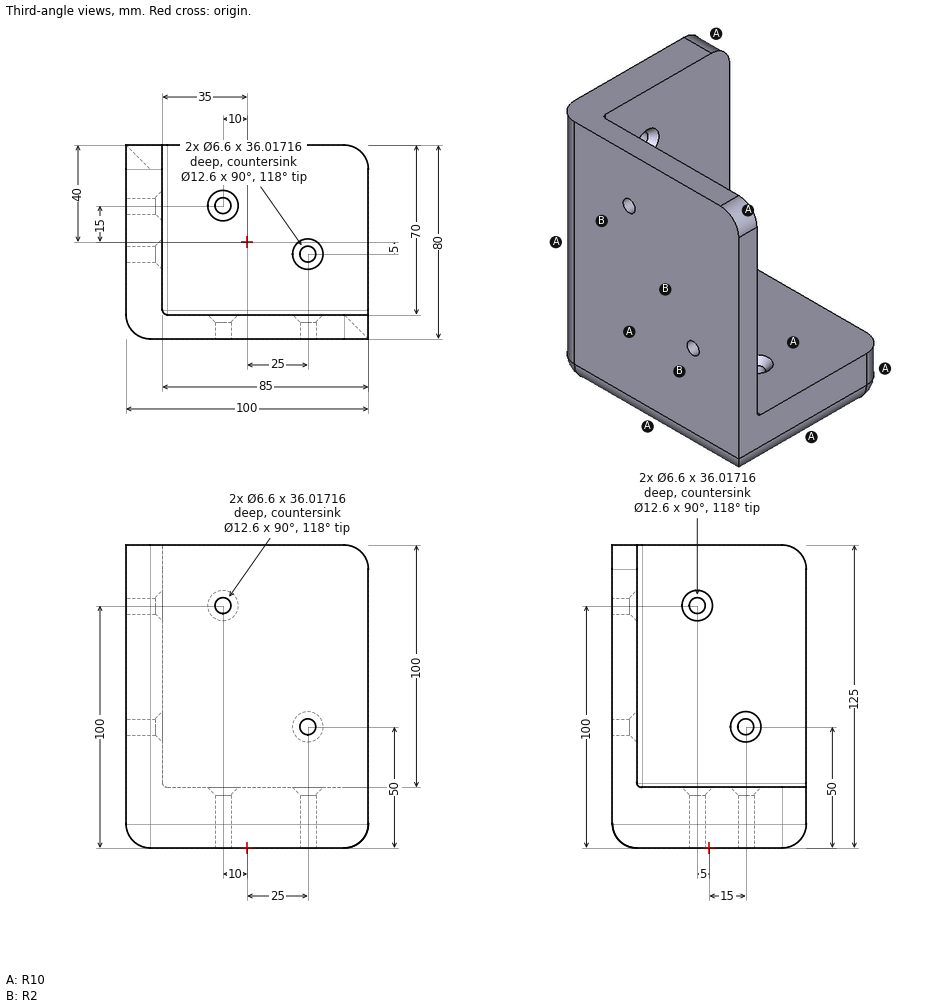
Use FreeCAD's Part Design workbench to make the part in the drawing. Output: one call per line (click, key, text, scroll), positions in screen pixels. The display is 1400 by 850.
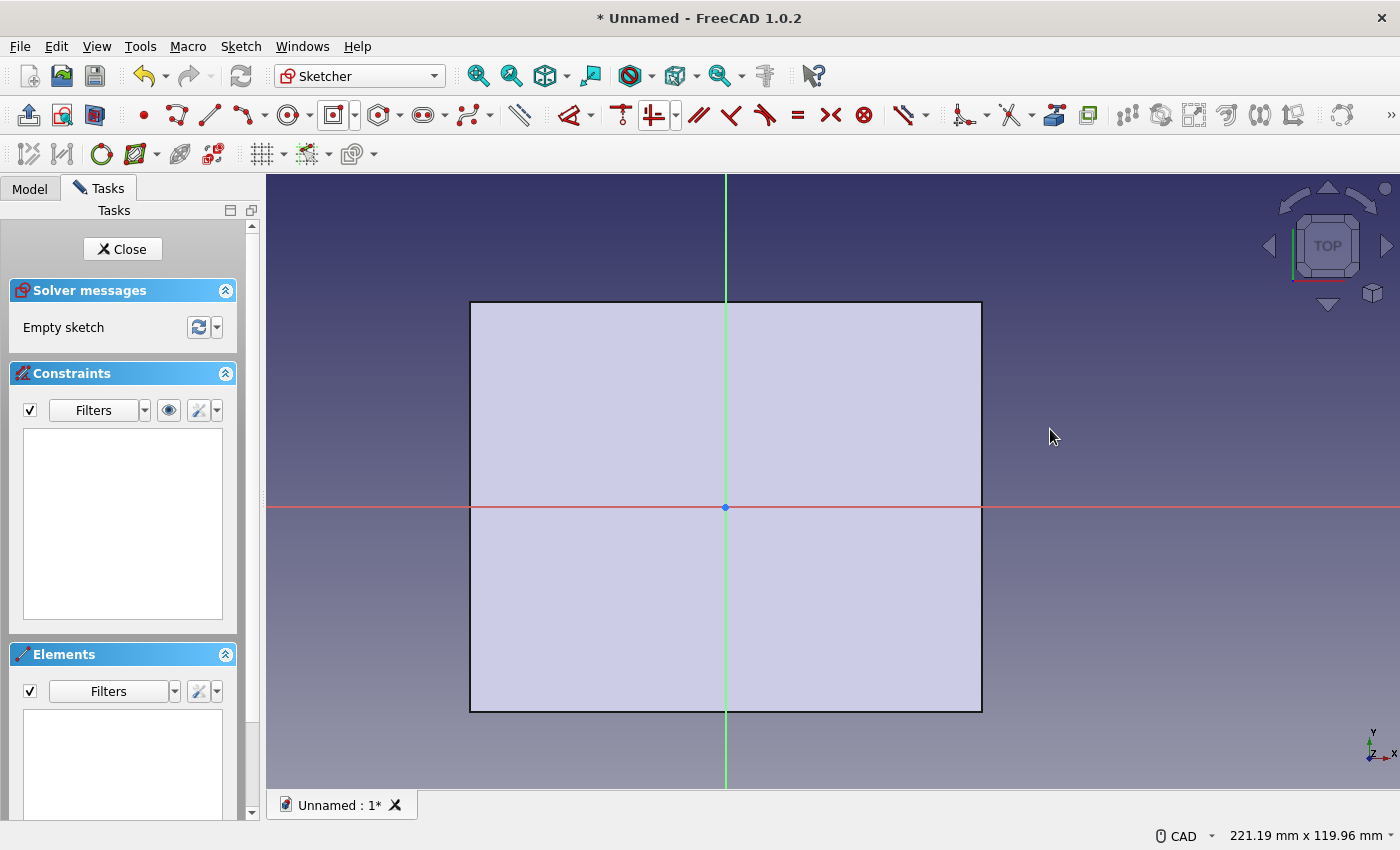
key(g)
key(r)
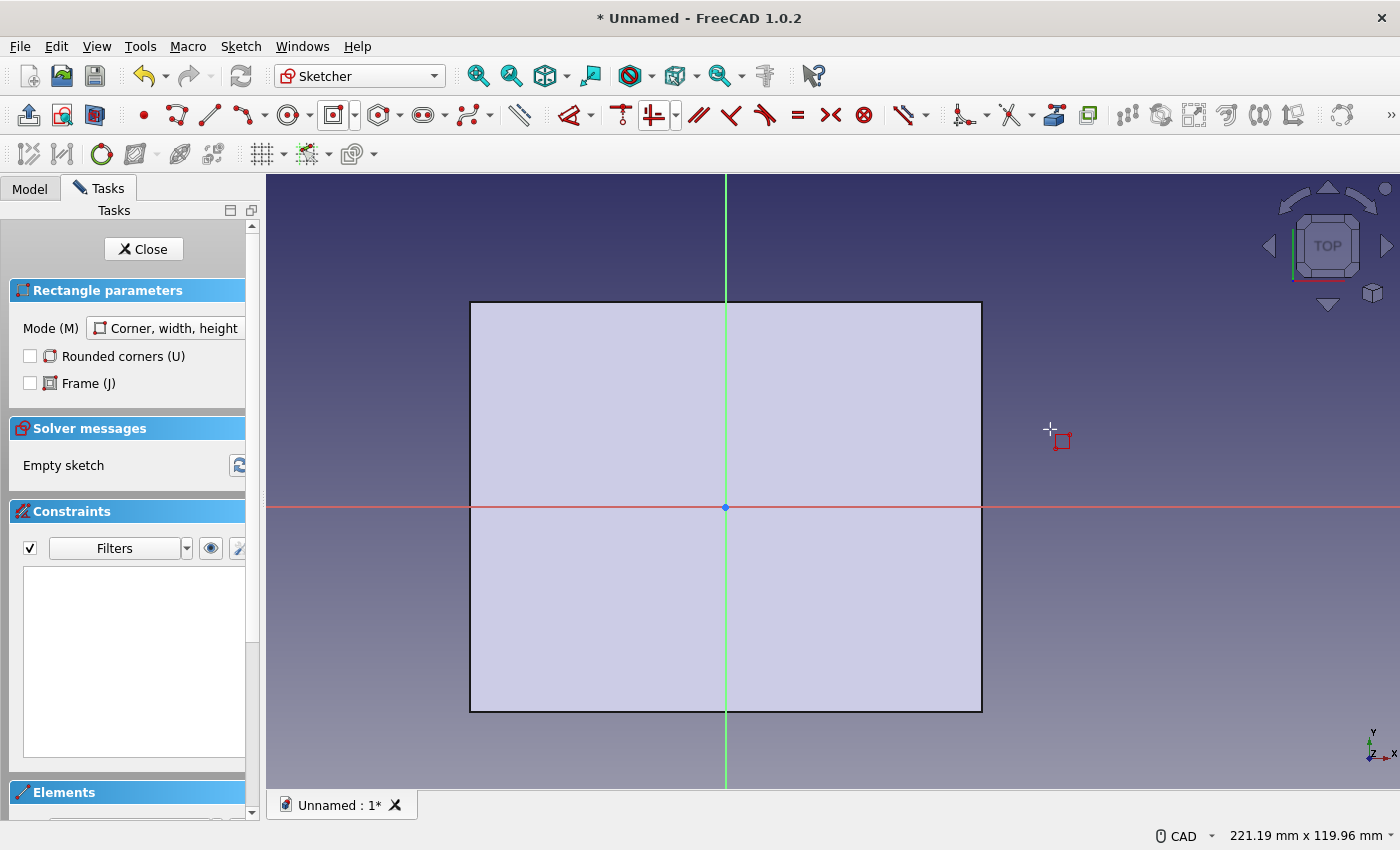
click(546, 302)
move(982, 661)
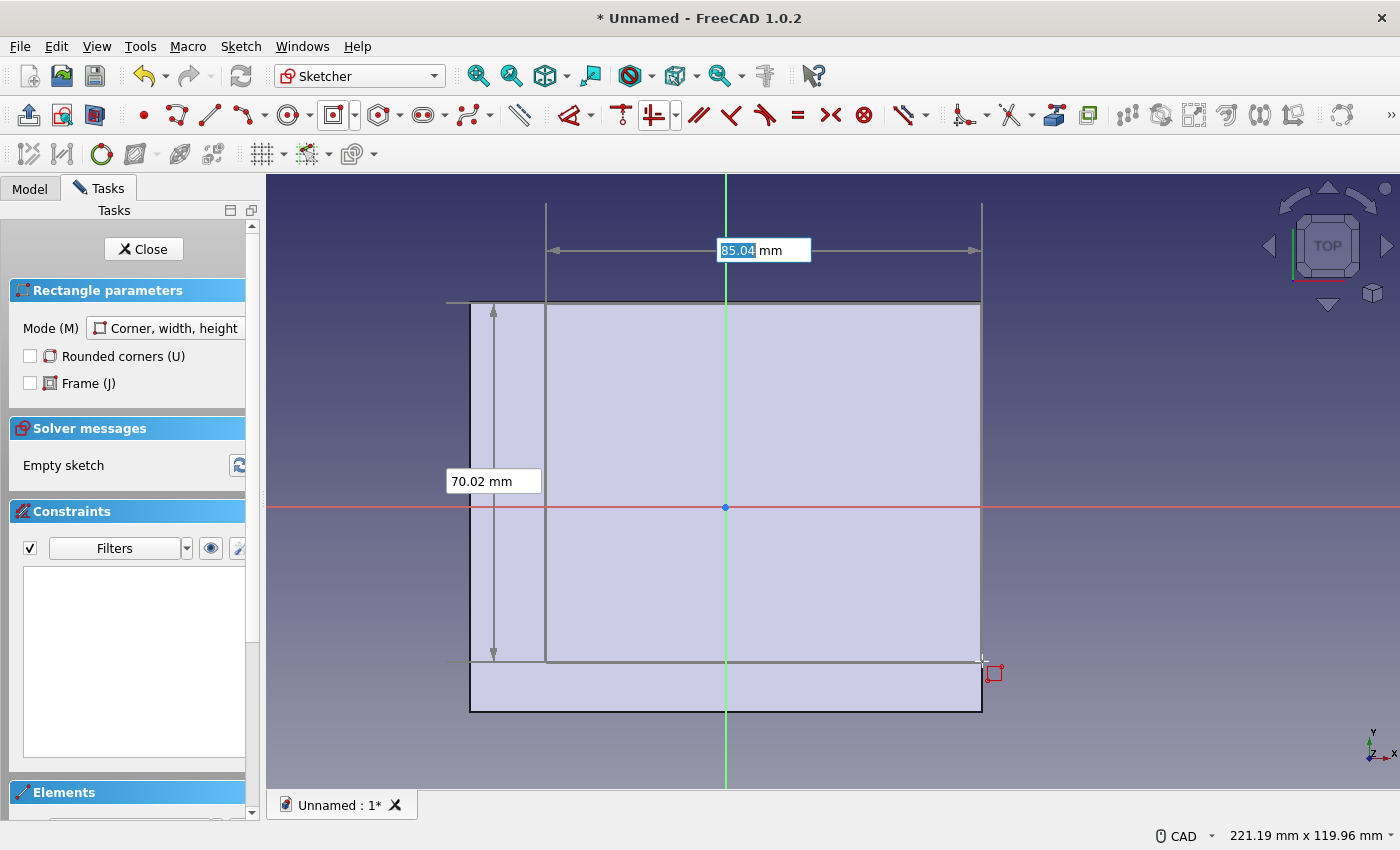
text(85)
key(Tab)
text(70)
key(Return)
key(Escape)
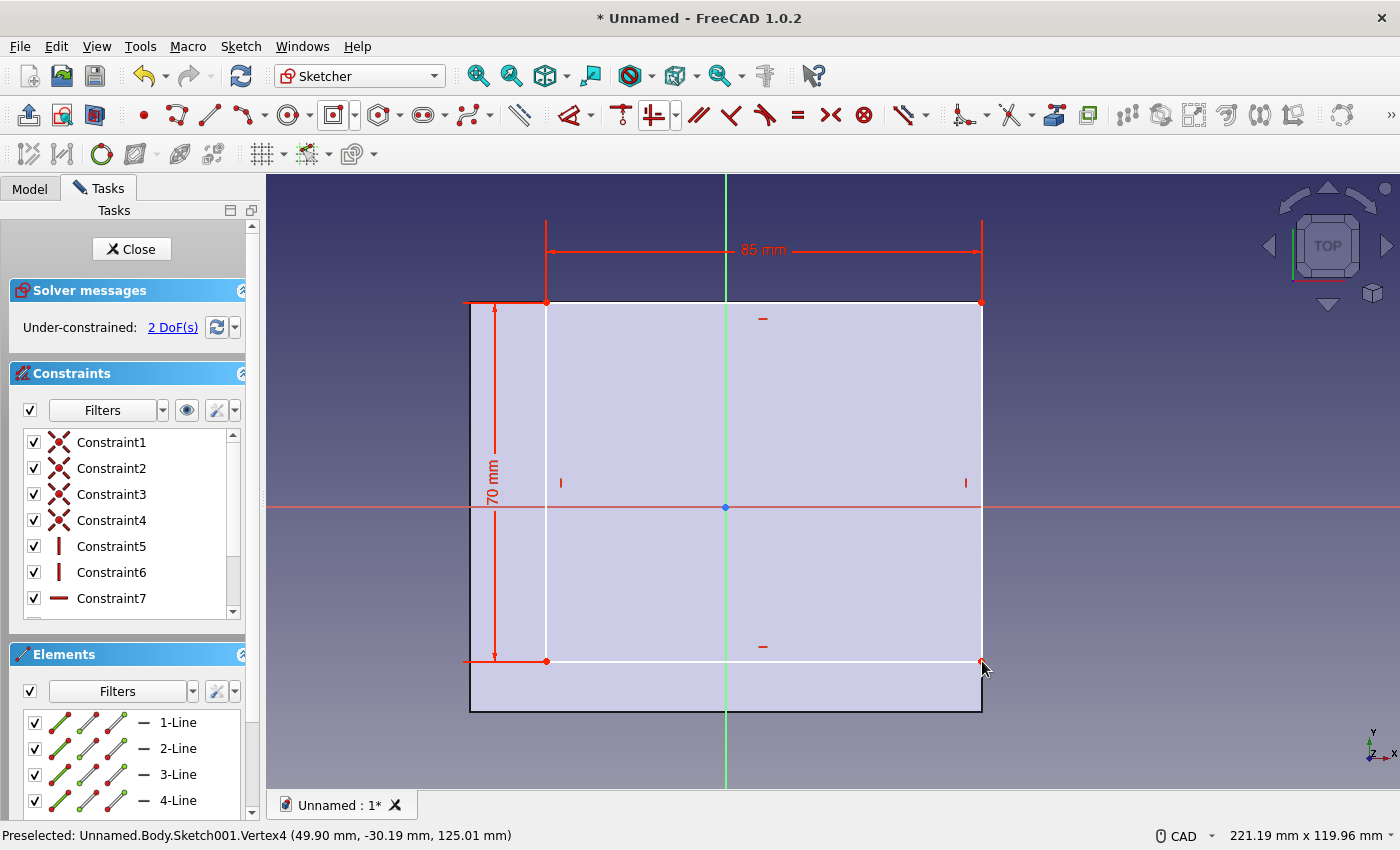
click(568, 116)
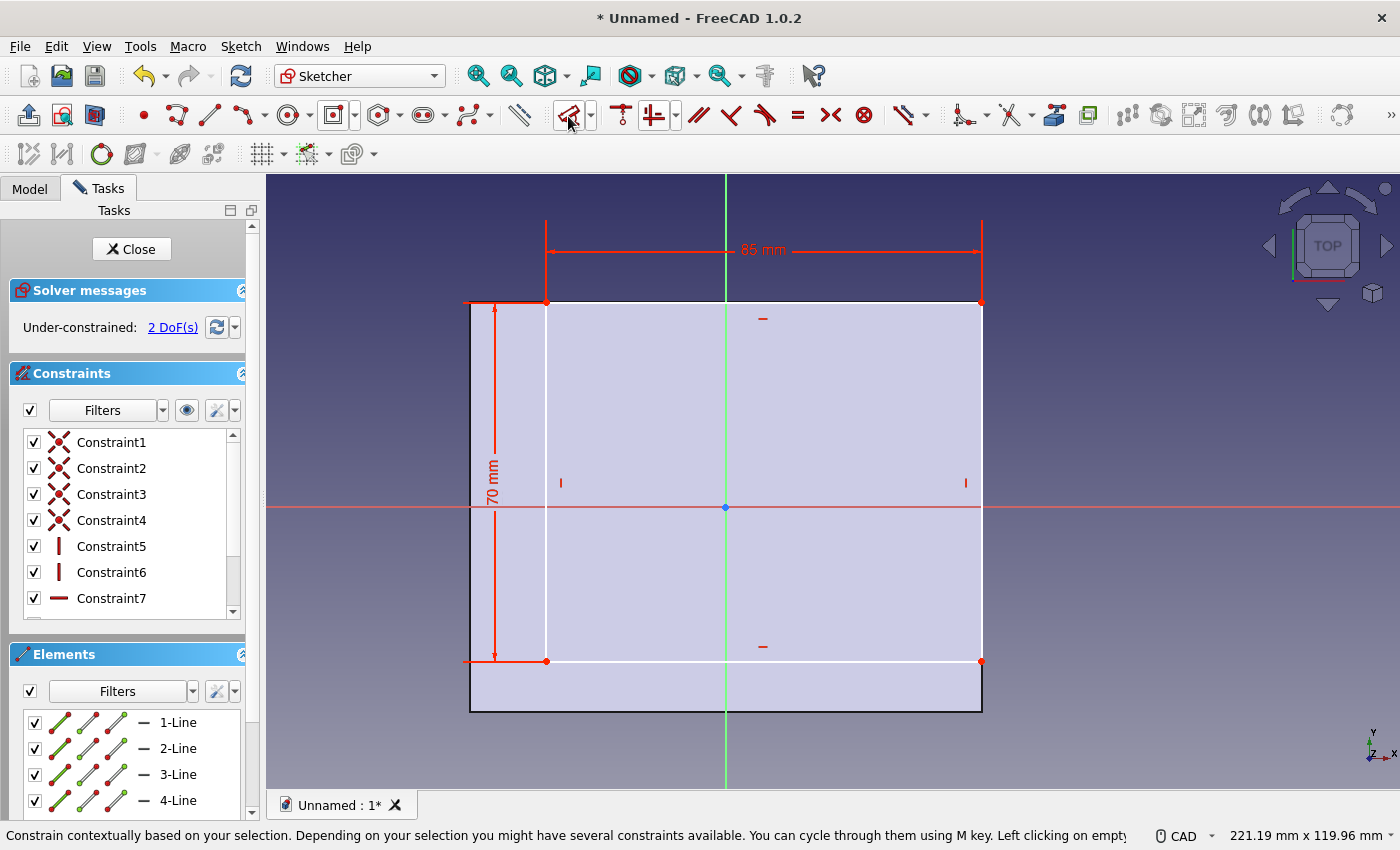
click(546, 303)
click(636, 269)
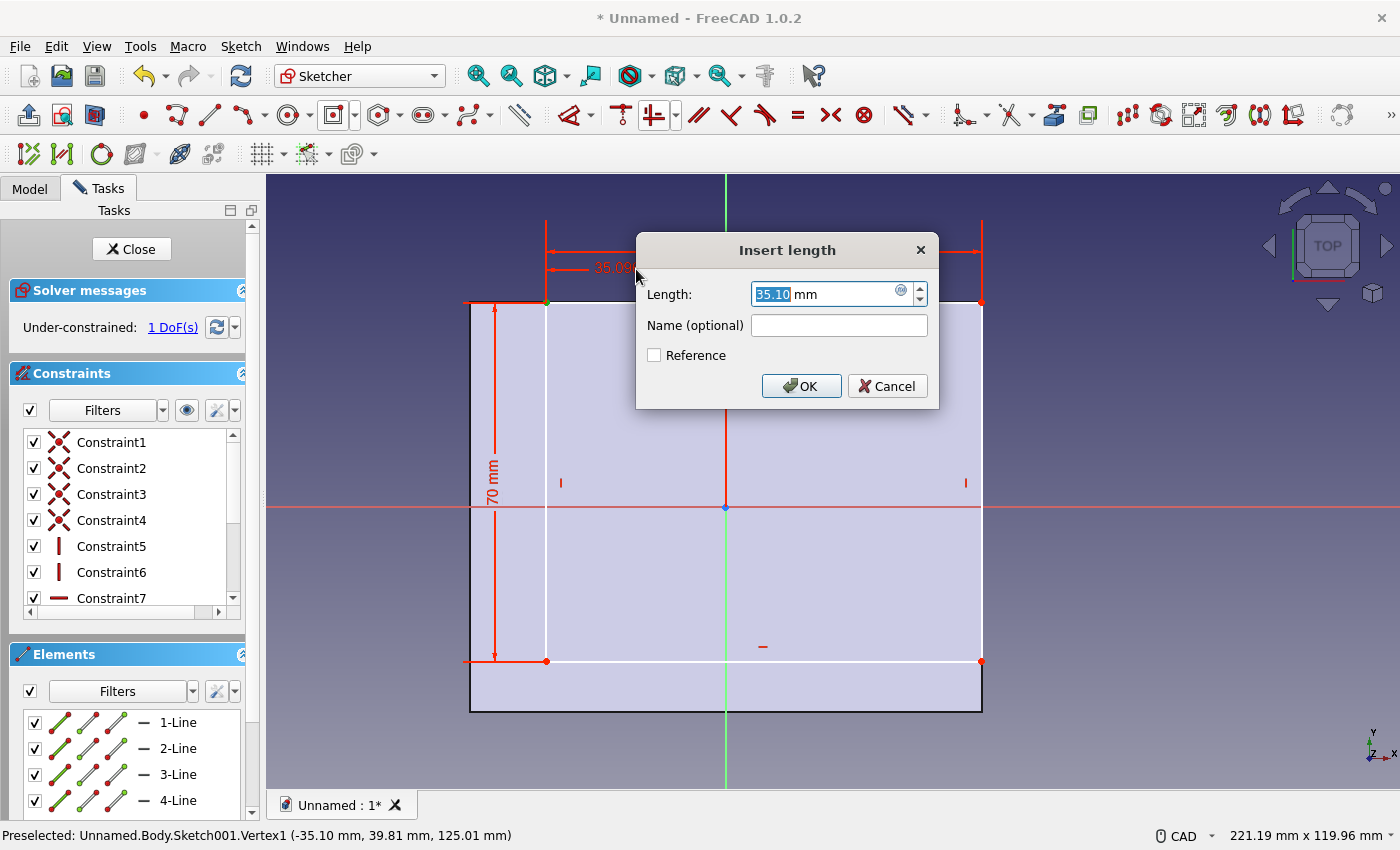
text(35)
key(Return)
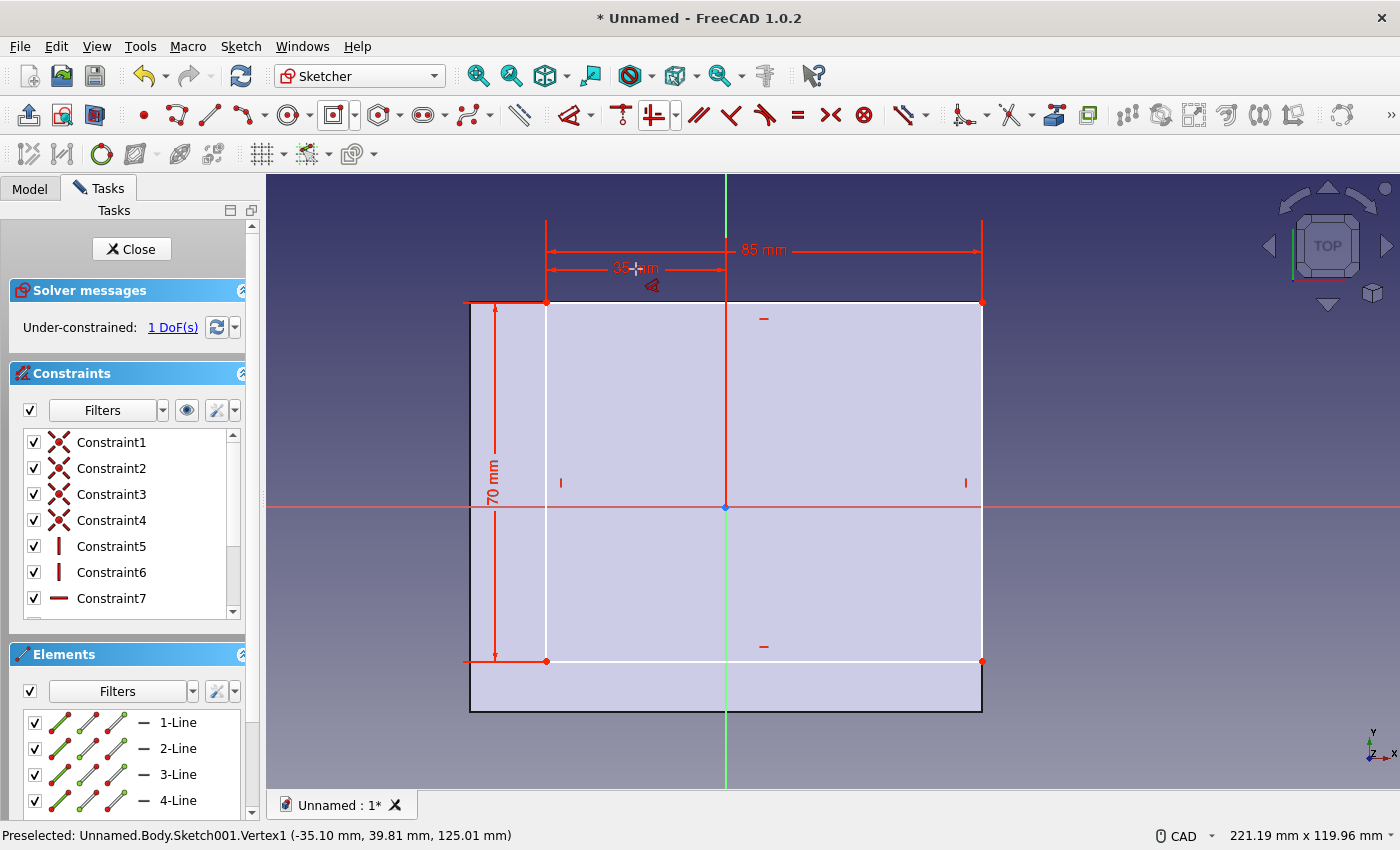
click(546, 303)
click(512, 405)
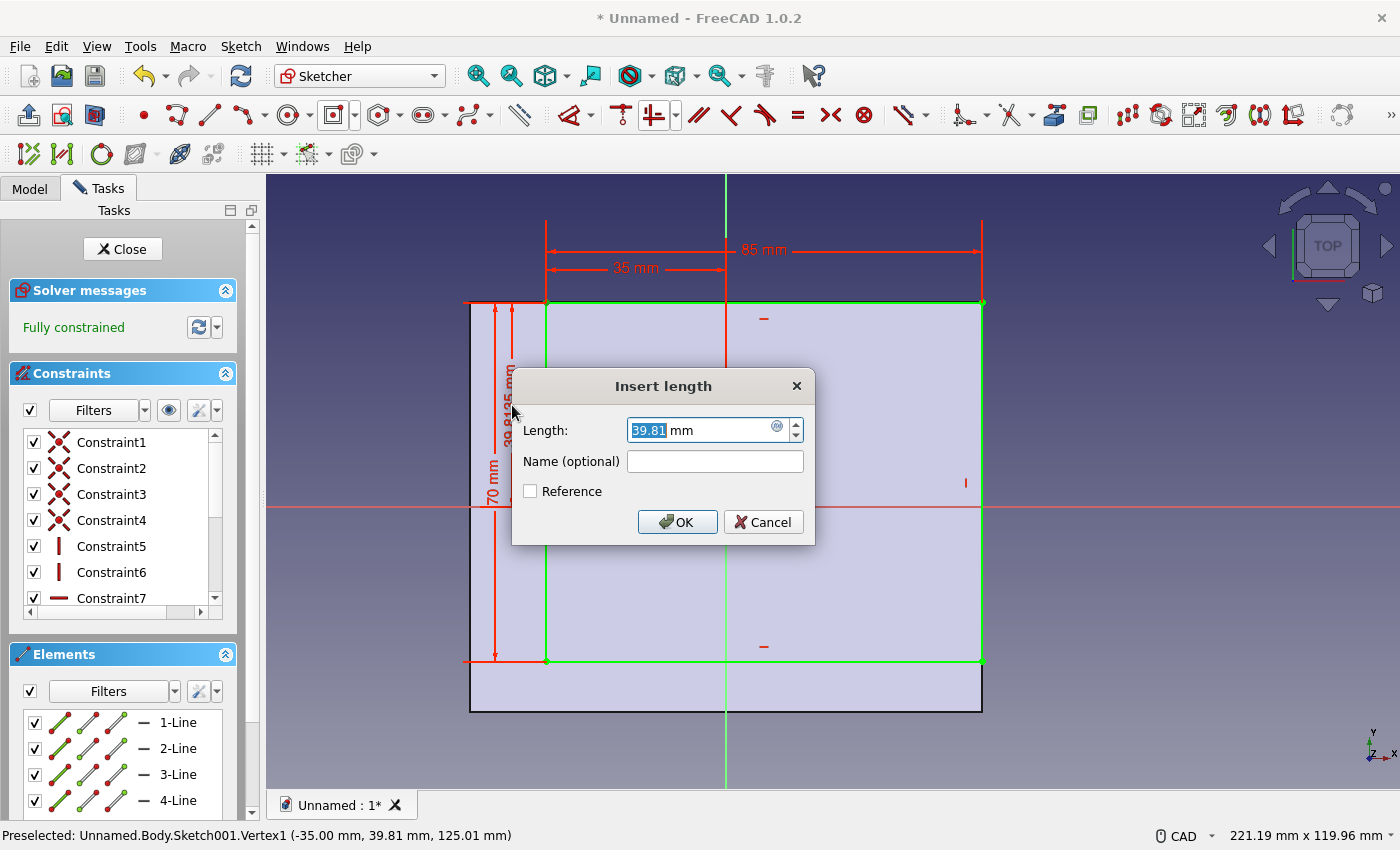
text(40)
key(Return)
key(Escape)